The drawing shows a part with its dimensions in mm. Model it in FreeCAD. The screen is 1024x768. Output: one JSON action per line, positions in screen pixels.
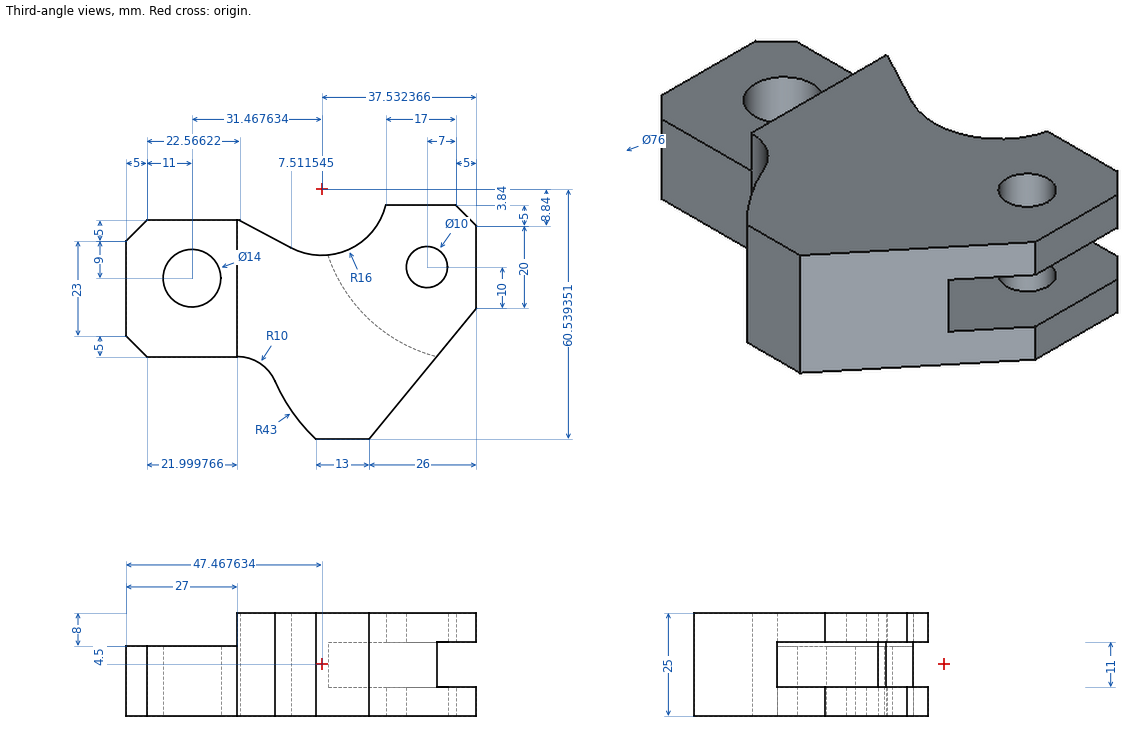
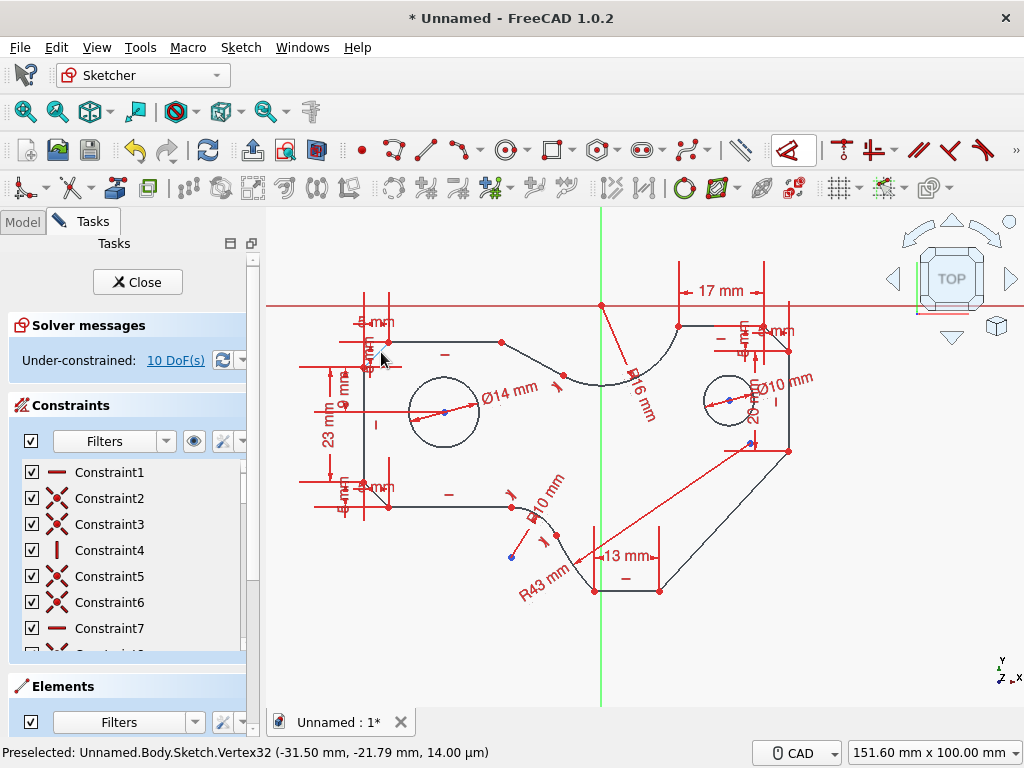
{"action": "left_click", "coordinate": [764, 326]}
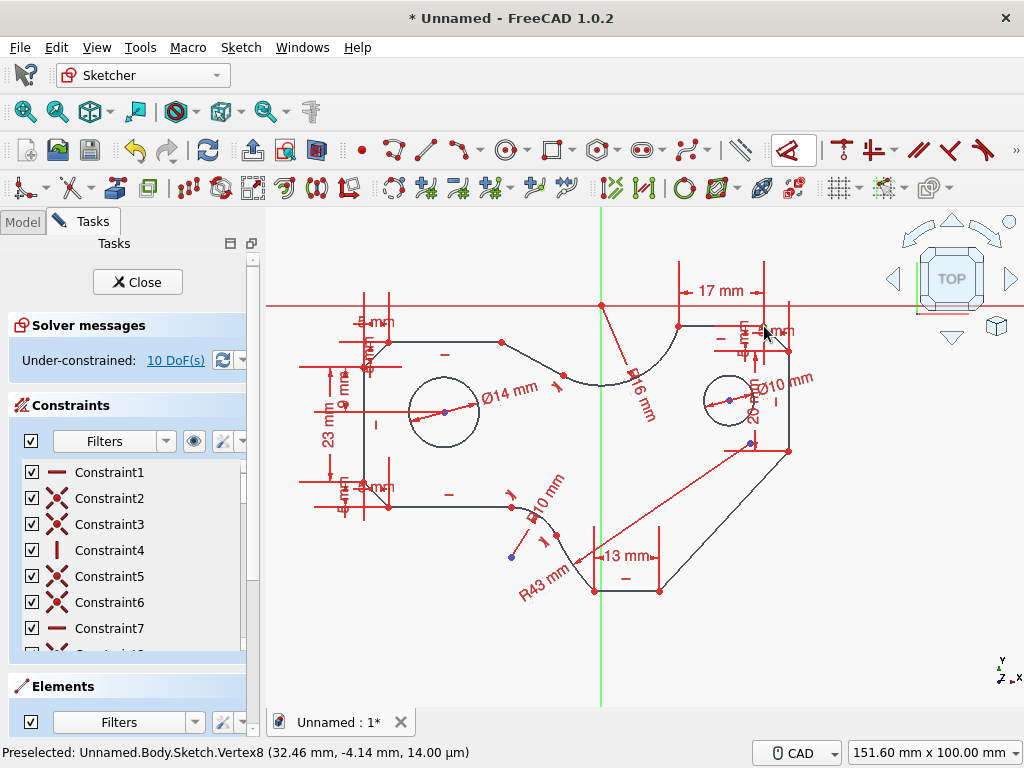
{"action": "left_click", "coordinate": [729, 401]}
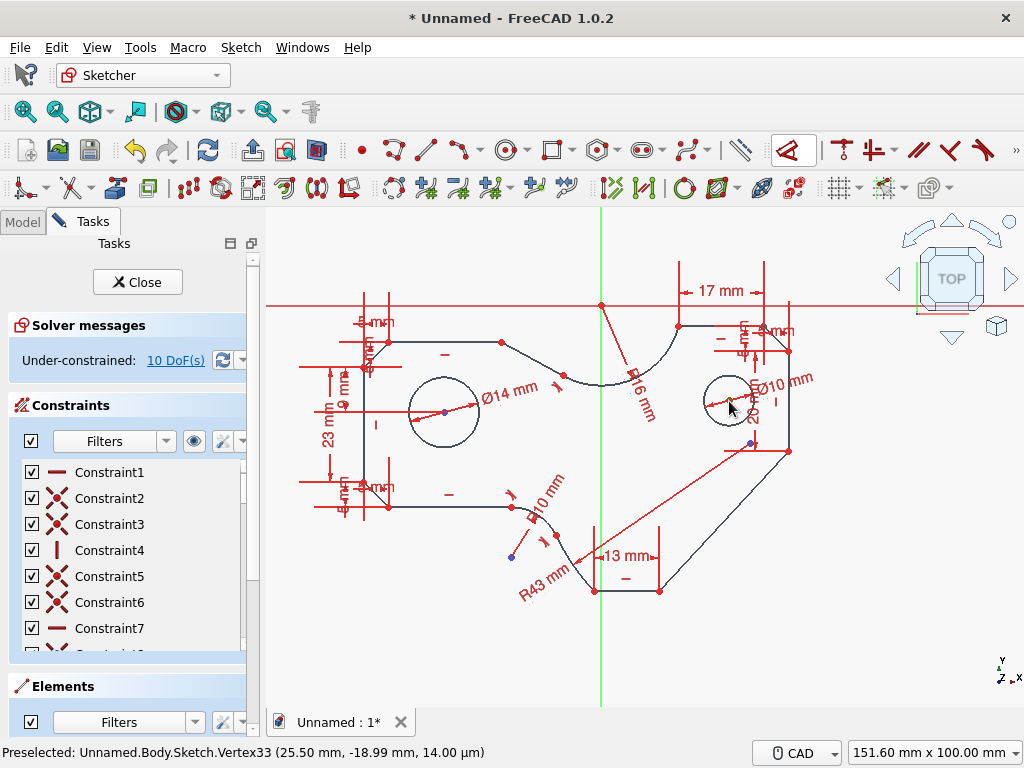
{"action": "left_click", "coordinate": [810, 150]}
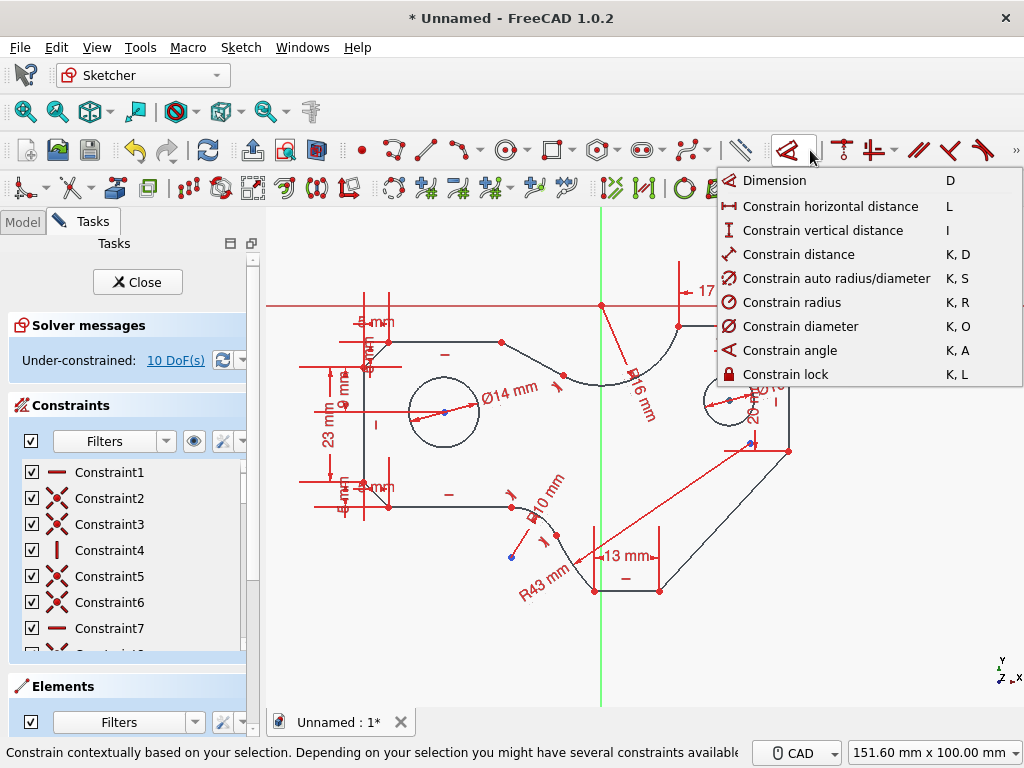
{"action": "left_click", "coordinate": [870, 206]}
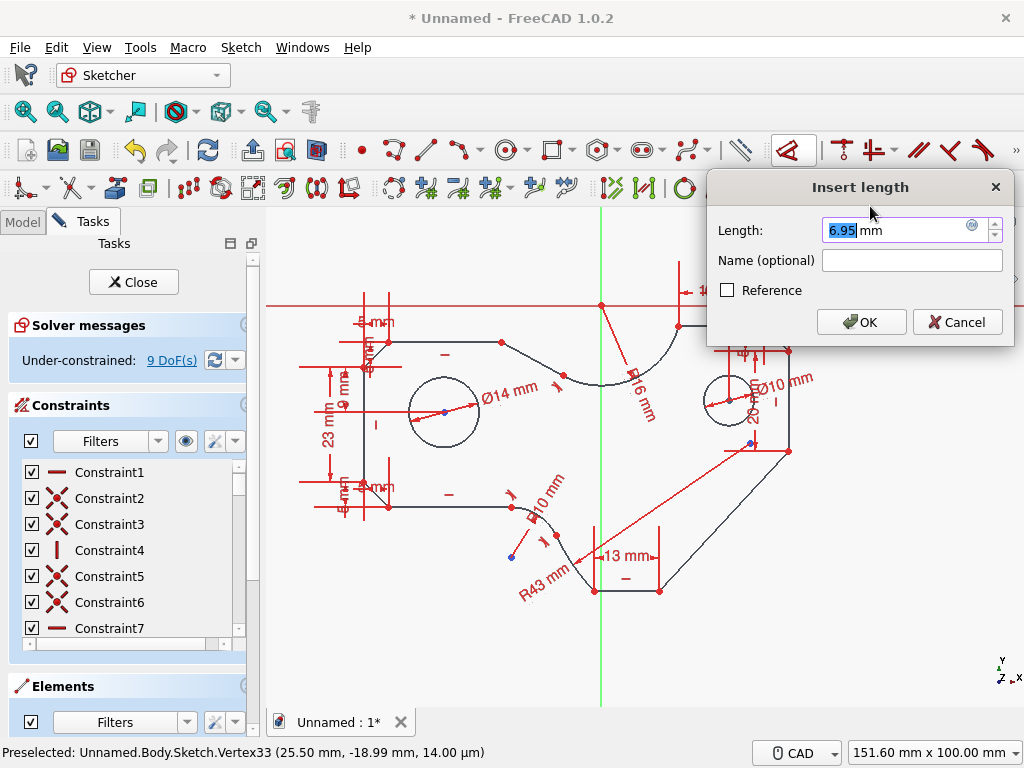
{"action": "type", "text": "7"}
{"action": "key", "text": "Return"}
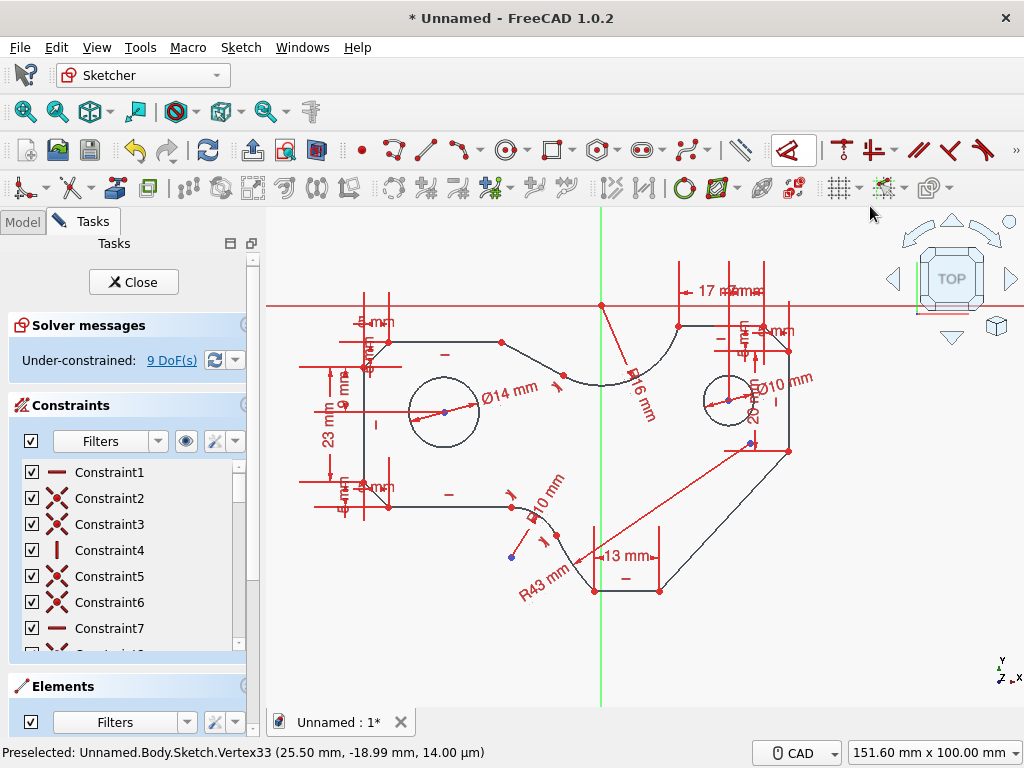
{"action": "left_click", "coordinate": [698, 549]}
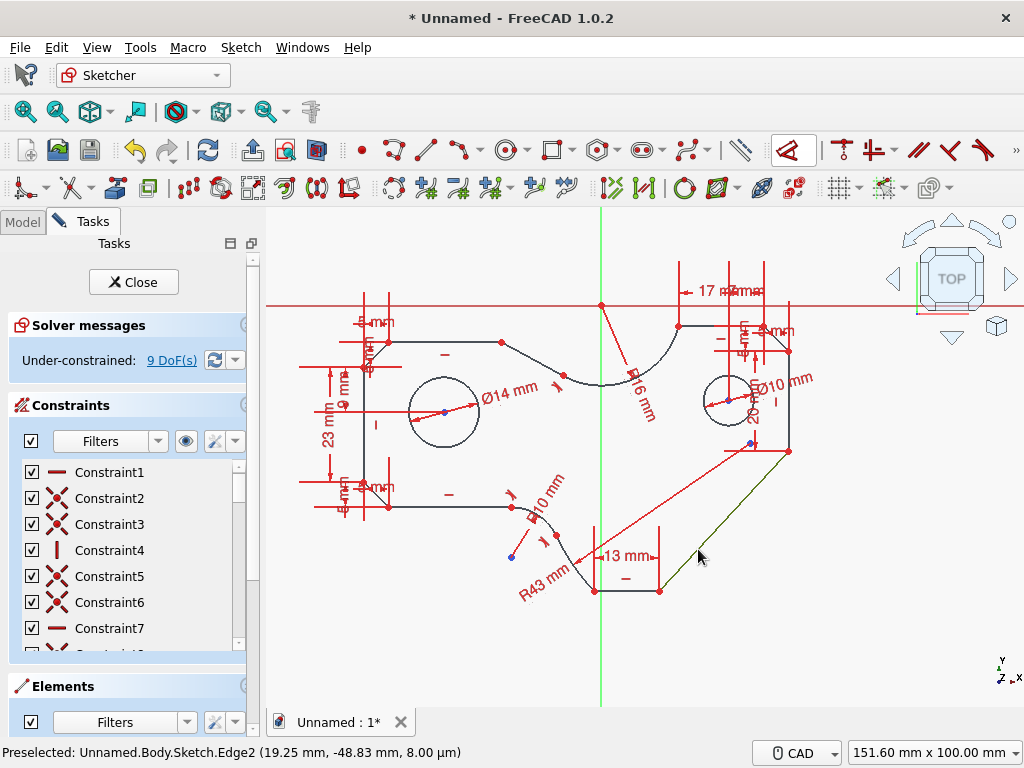
{"action": "key", "text": "l"}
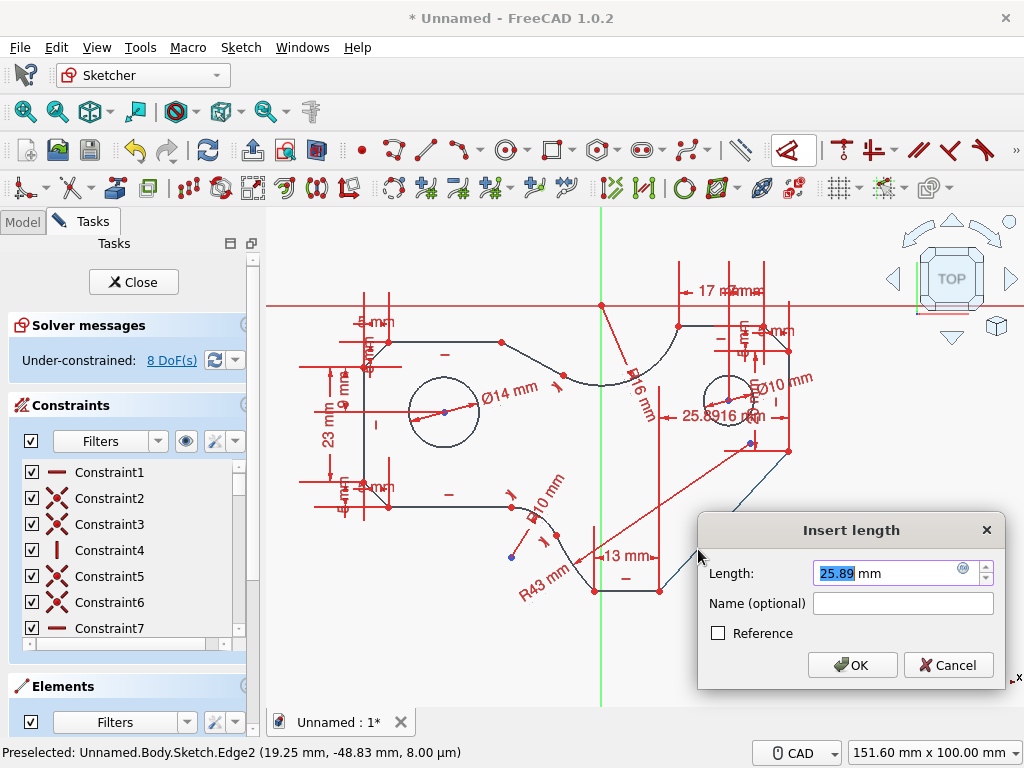
{"action": "type", "text": "26"}
{"action": "key", "text": "Return"}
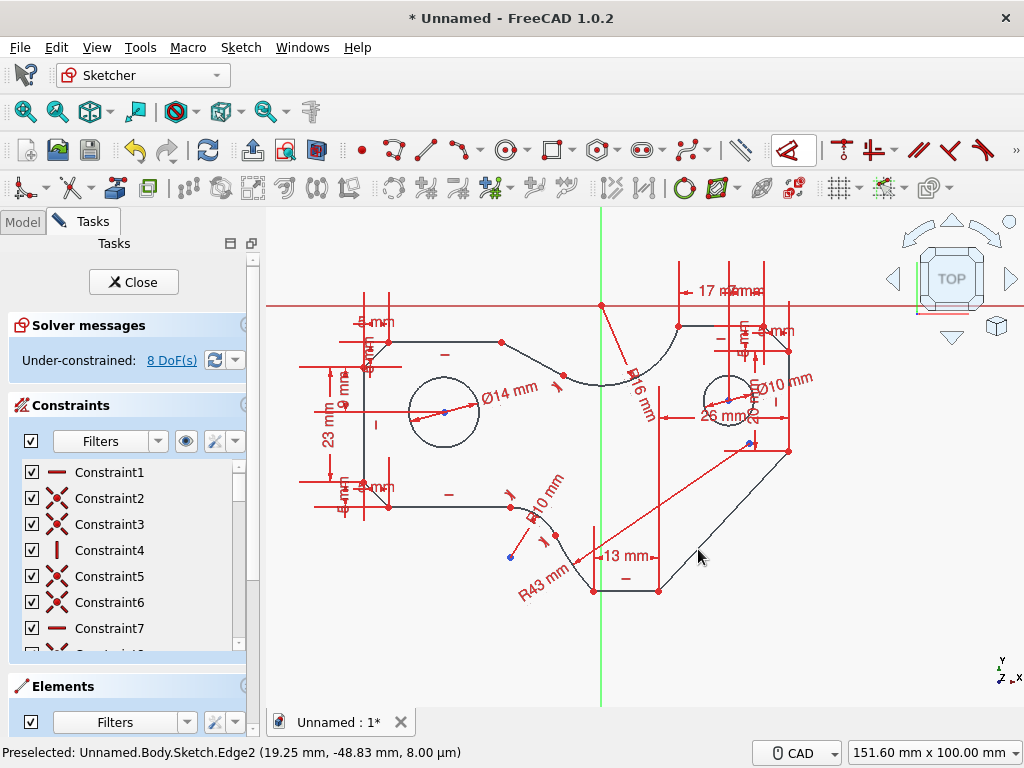
{"action": "left_click", "coordinate": [389, 342]}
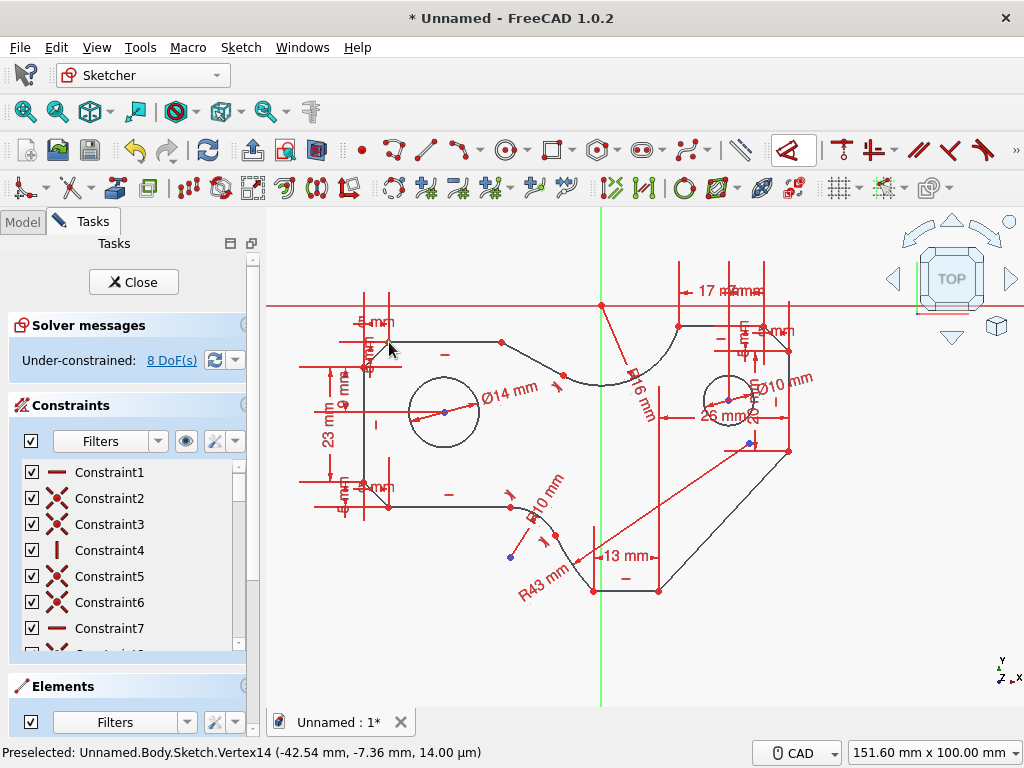
{"action": "left_click", "coordinate": [444, 412]}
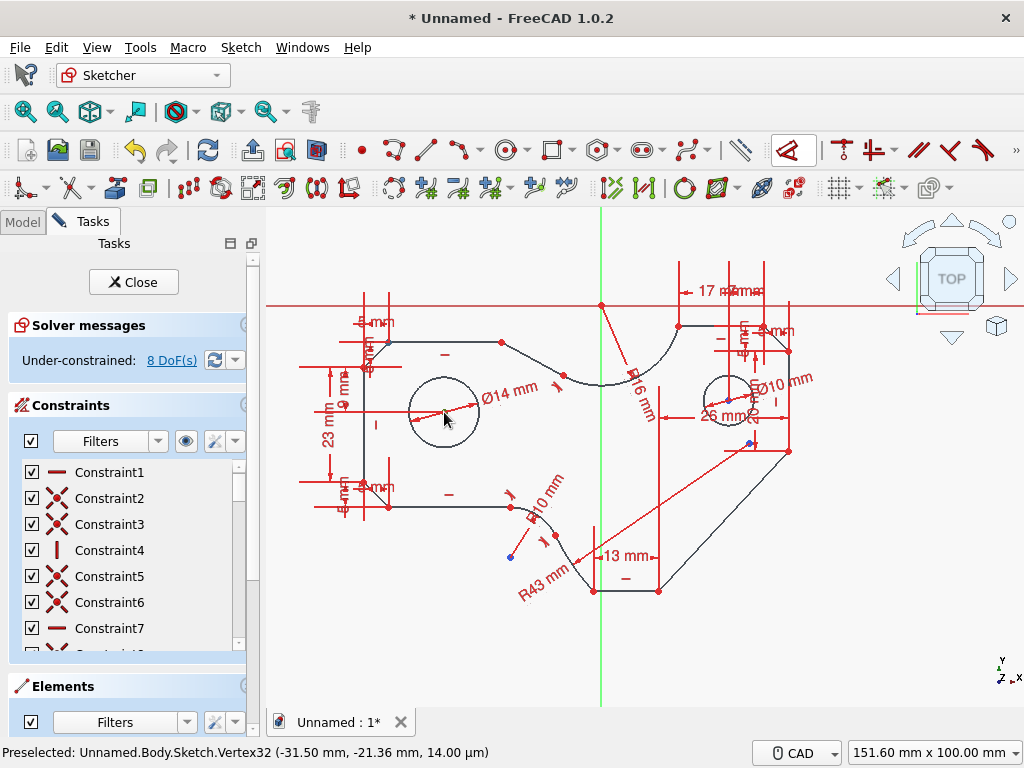
{"action": "left_click", "coordinate": [810, 150]}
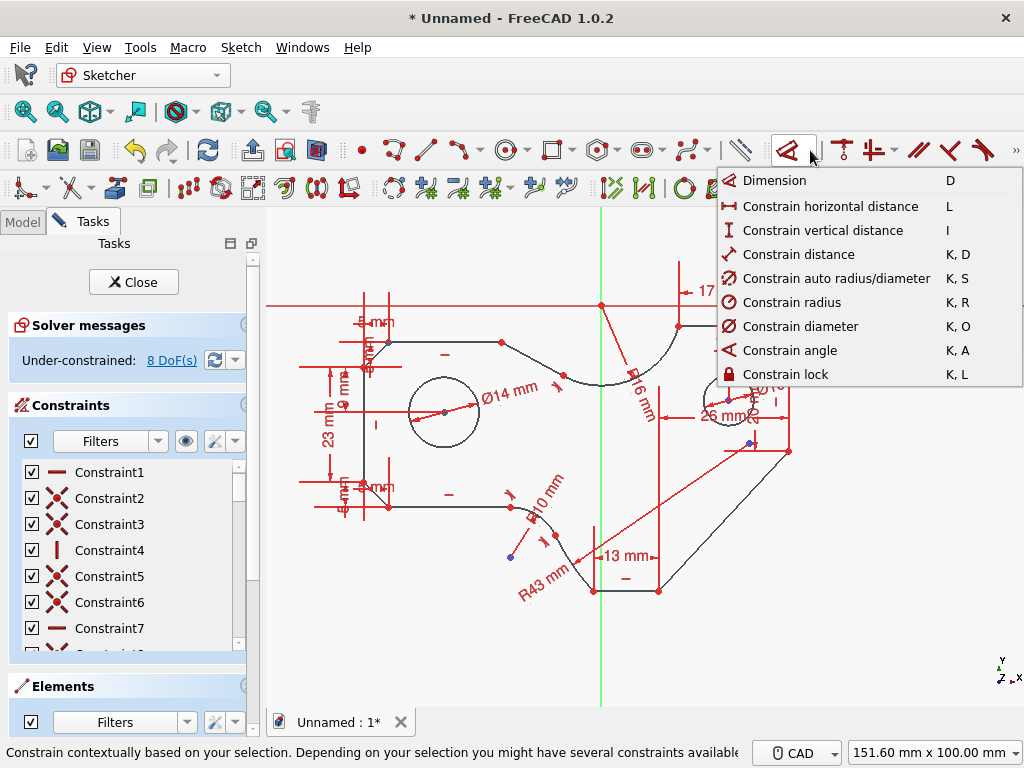
{"action": "left_click", "coordinate": [870, 206]}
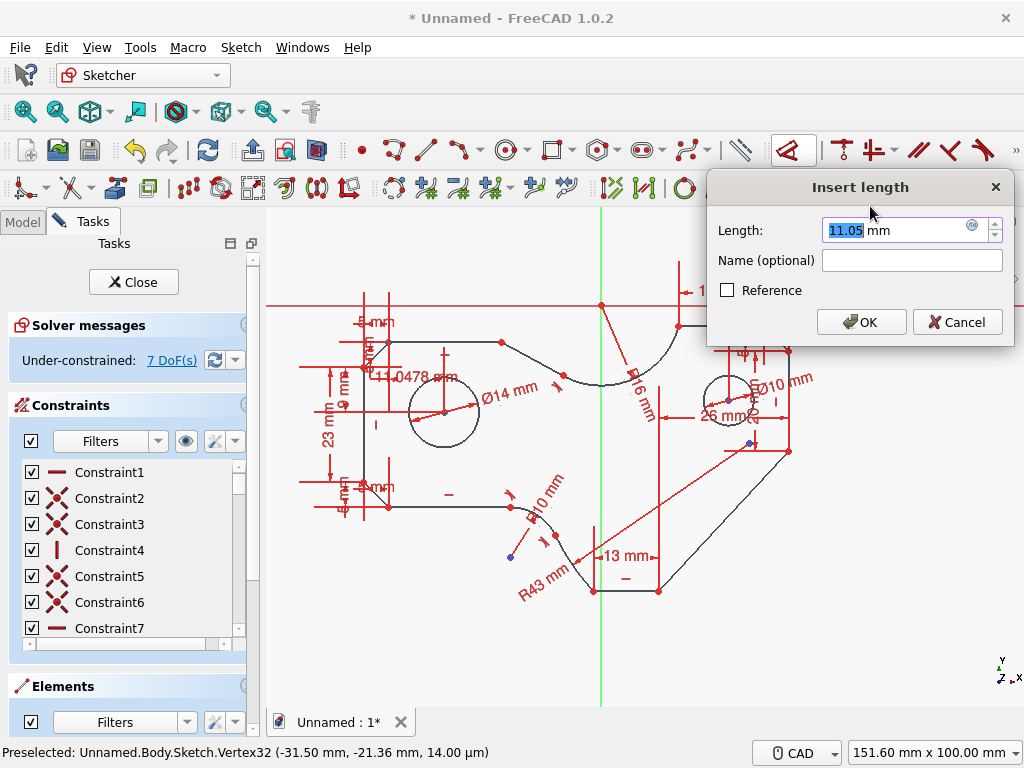
{"action": "type", "text": "11"}
{"action": "key", "text": "Return"}